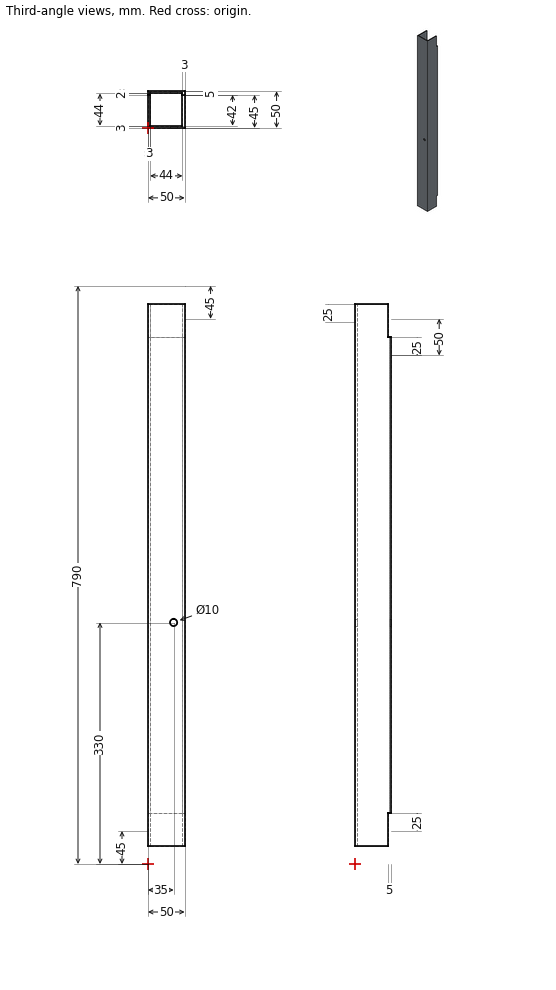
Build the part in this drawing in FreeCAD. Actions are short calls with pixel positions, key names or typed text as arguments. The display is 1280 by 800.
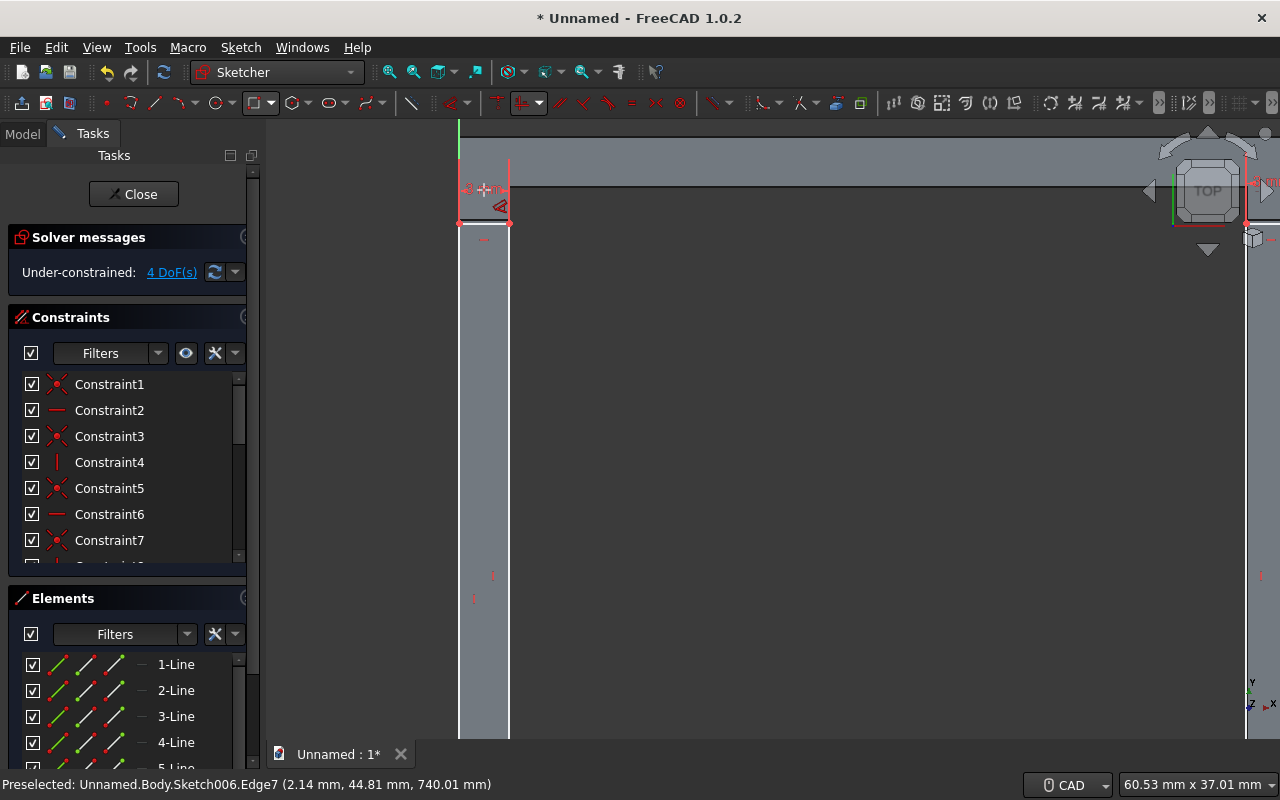
scroll(494, 224, down, 3)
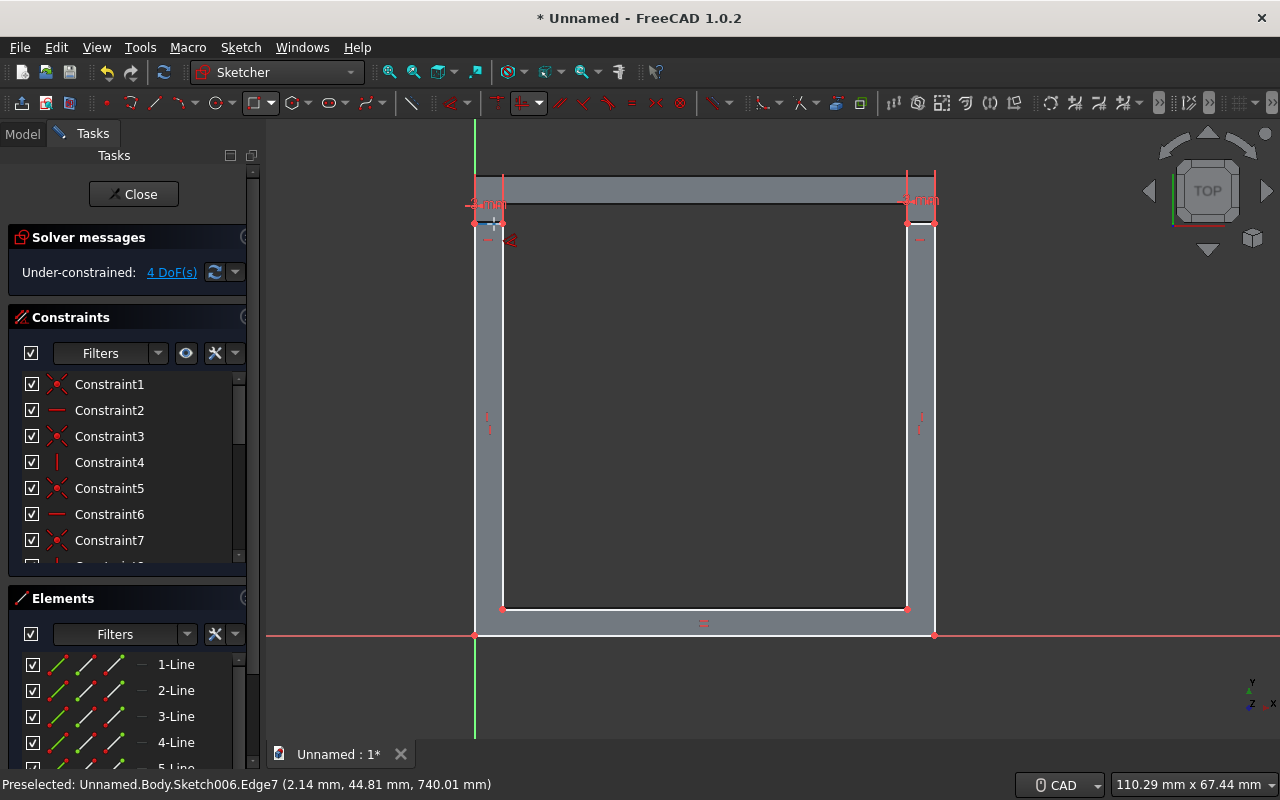
click(613, 636)
click(705, 670)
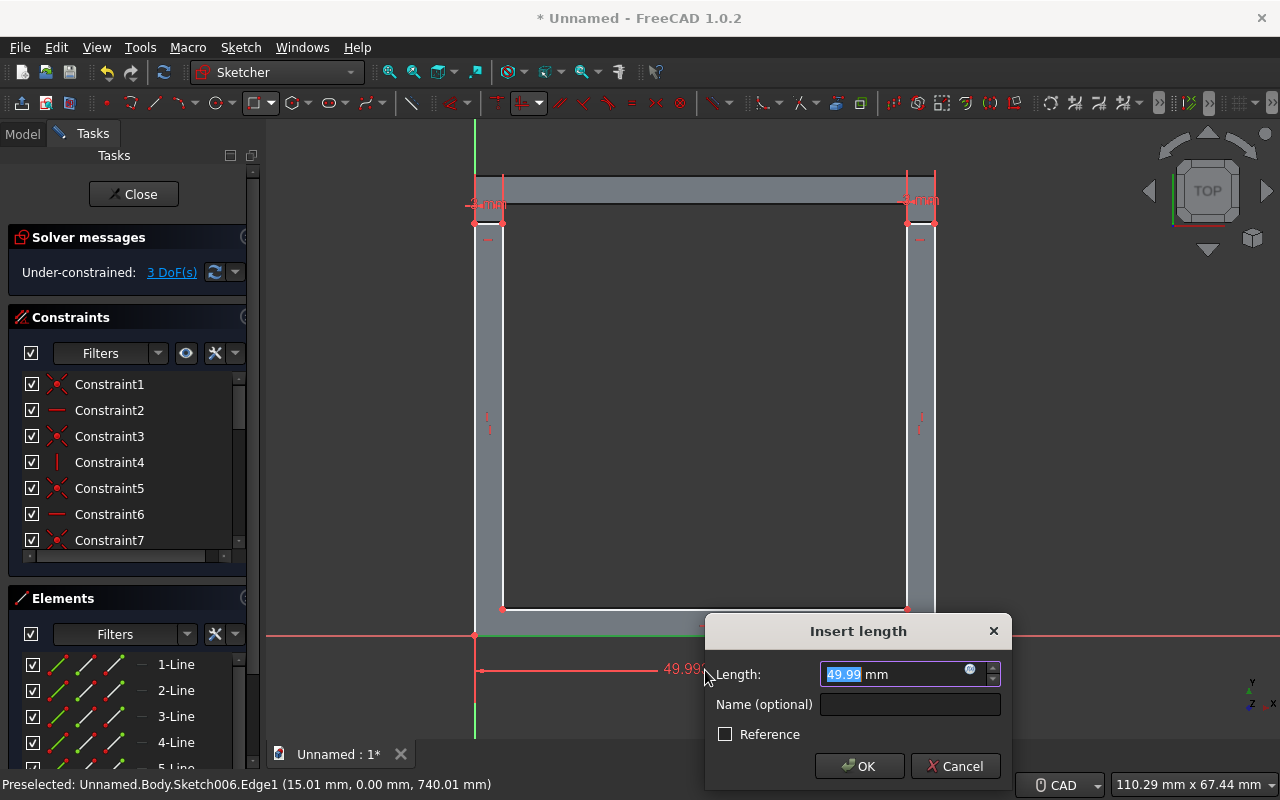
text(50)
key(Return)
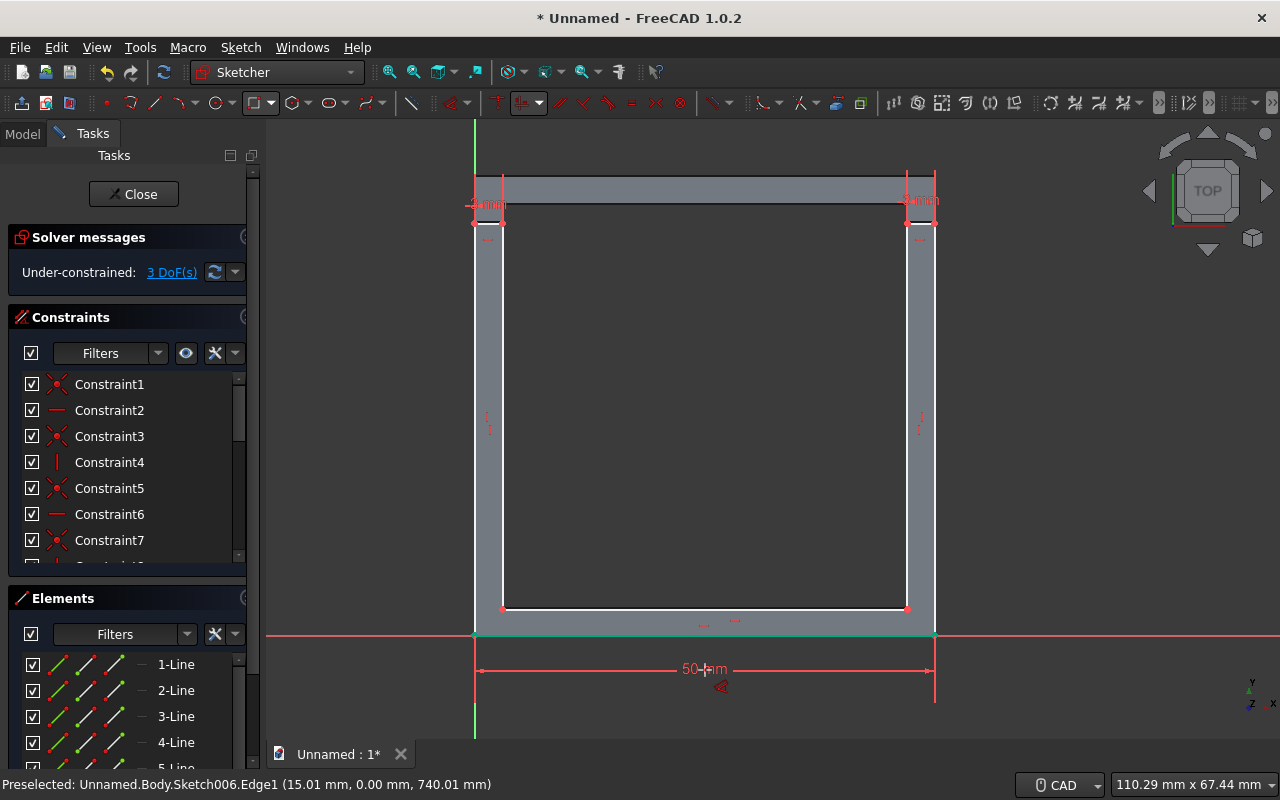
click(935, 512)
click(969, 430)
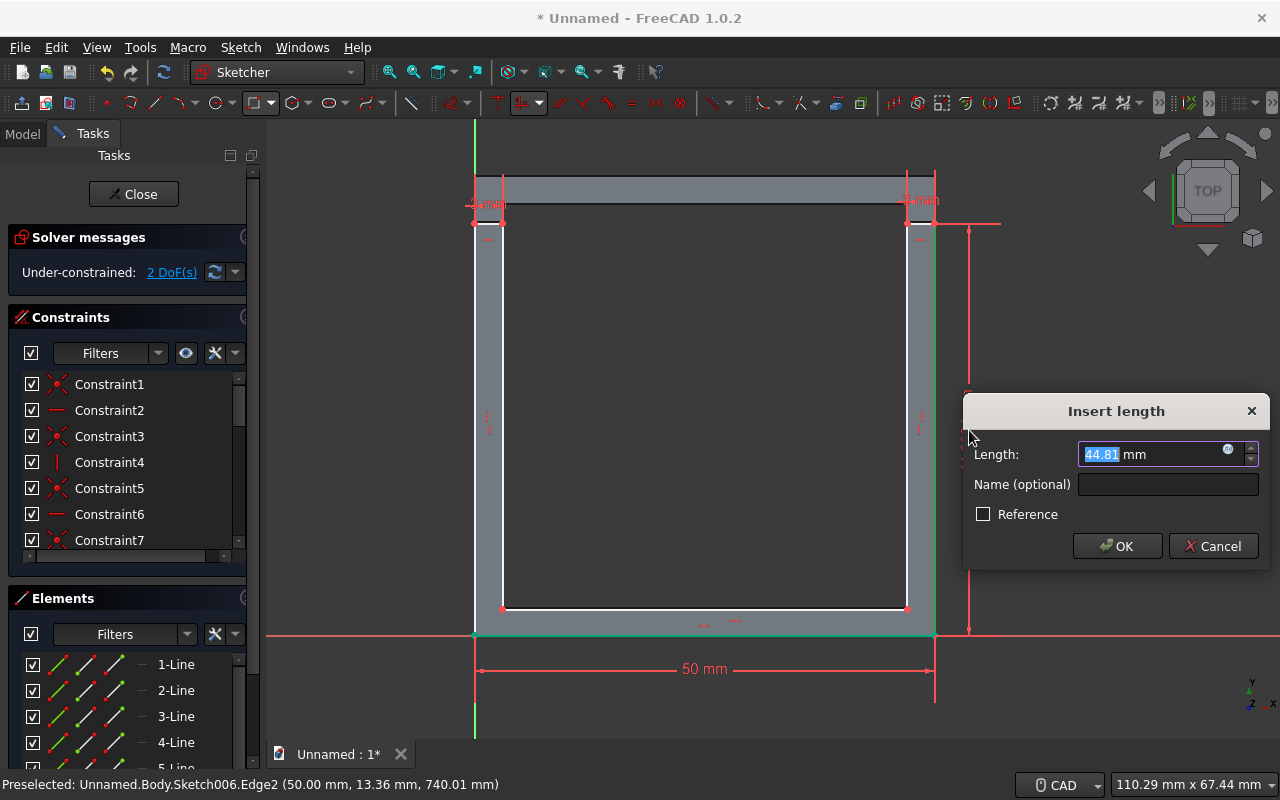
text(45)
key(Return)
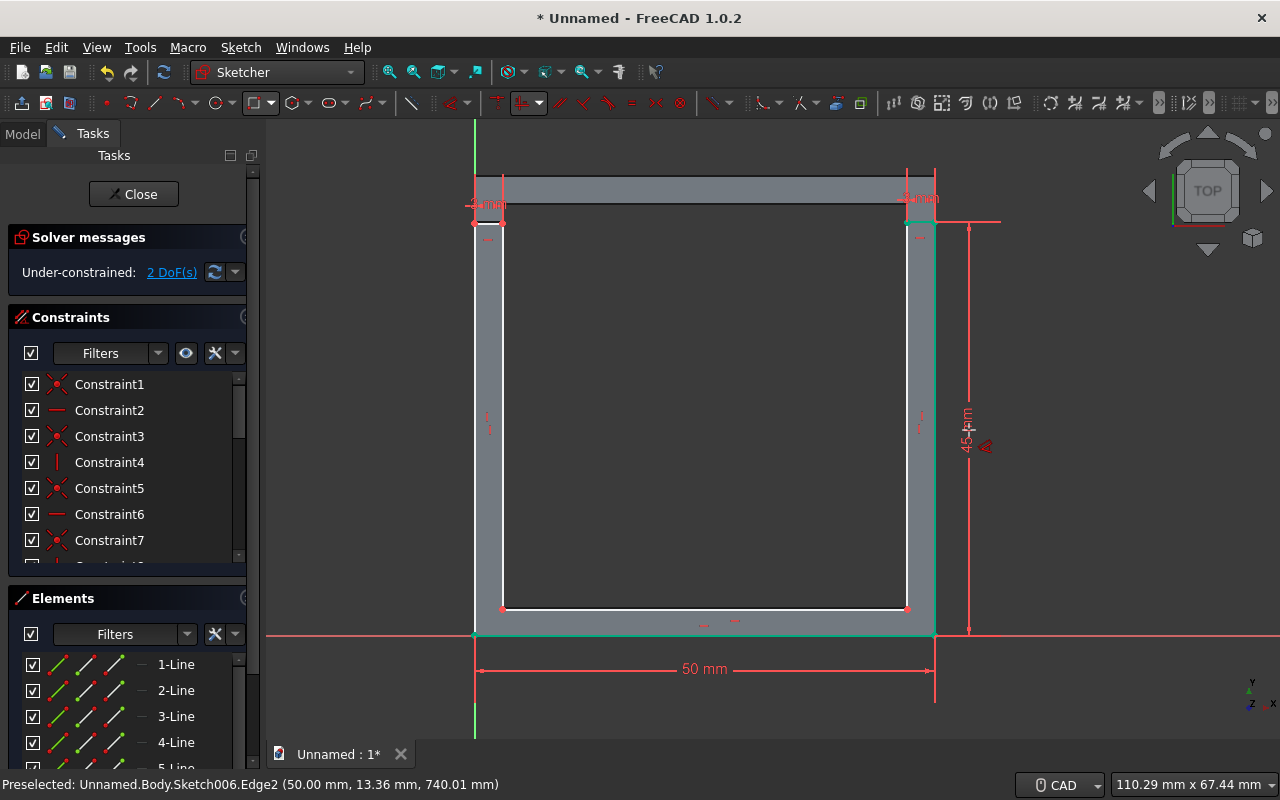
click(907, 338)
click(873, 416)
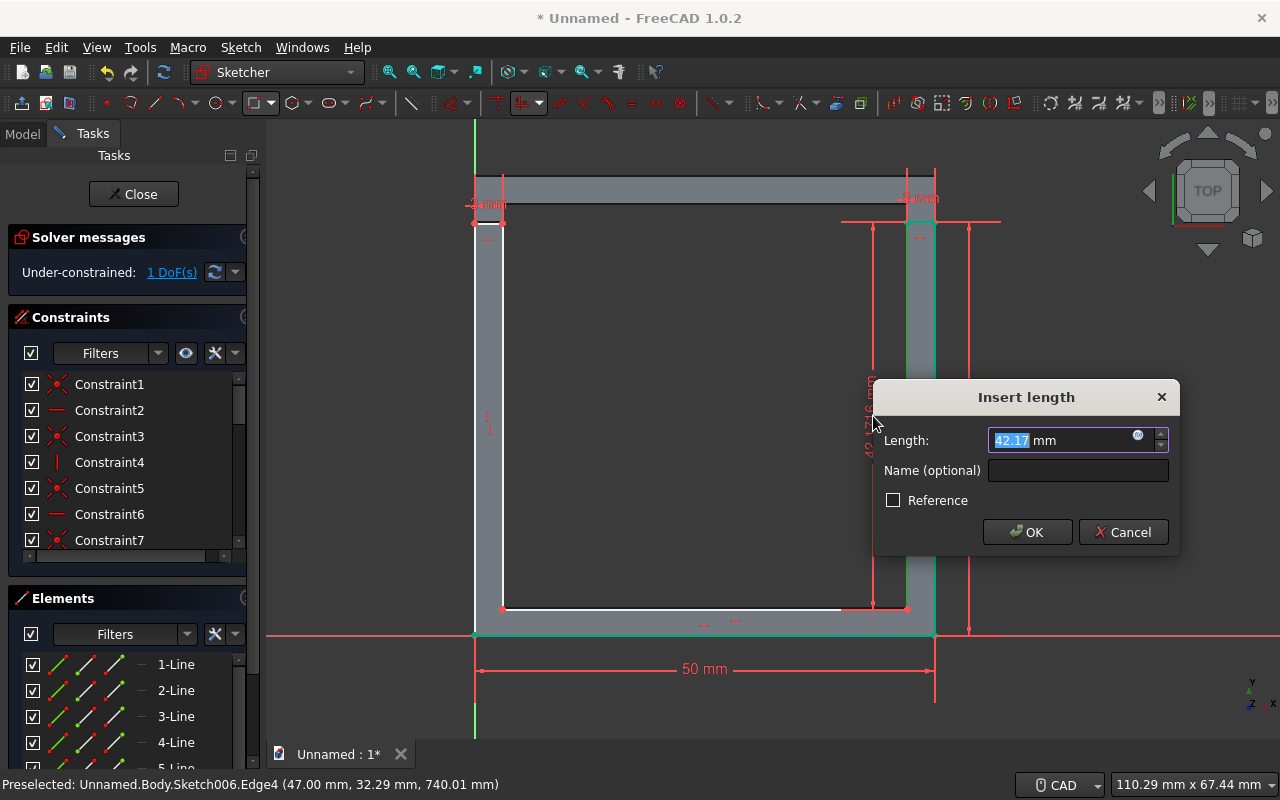
text(42)
key(Return)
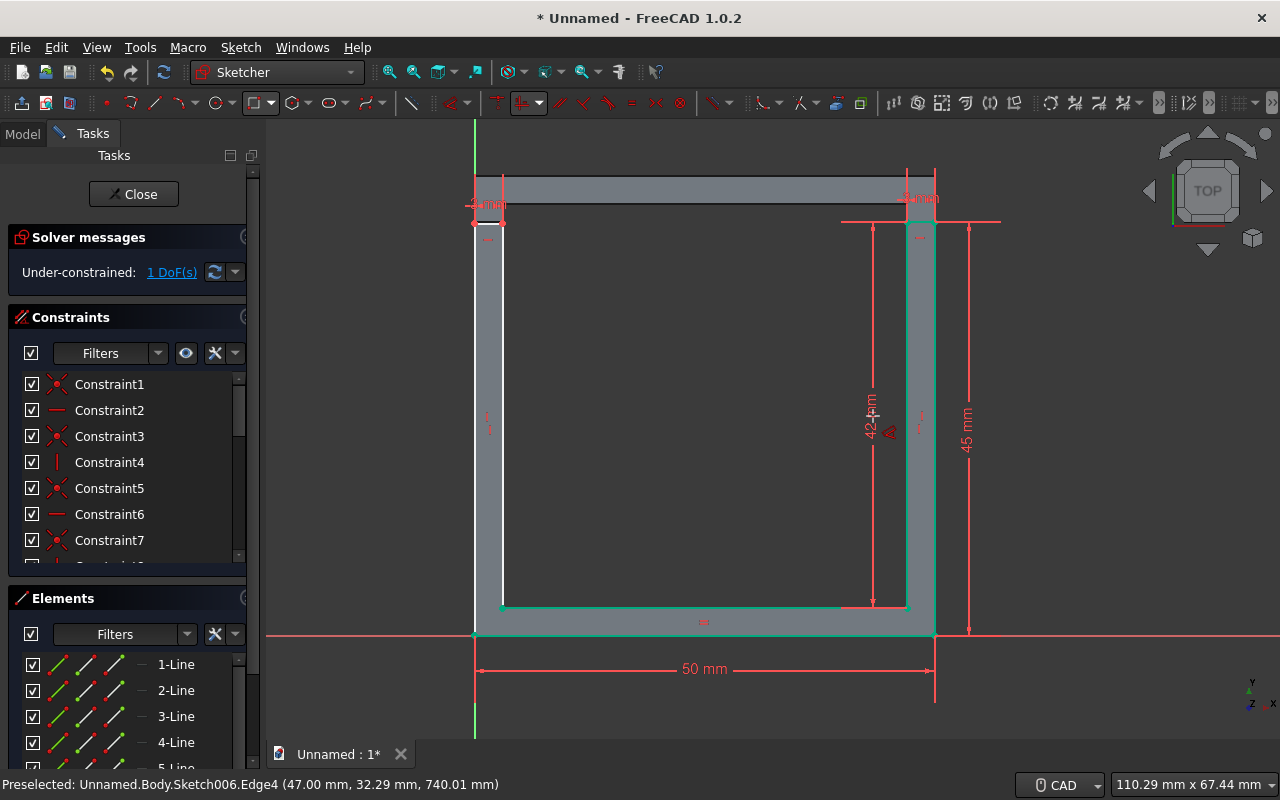
click(503, 493)
click(537, 416)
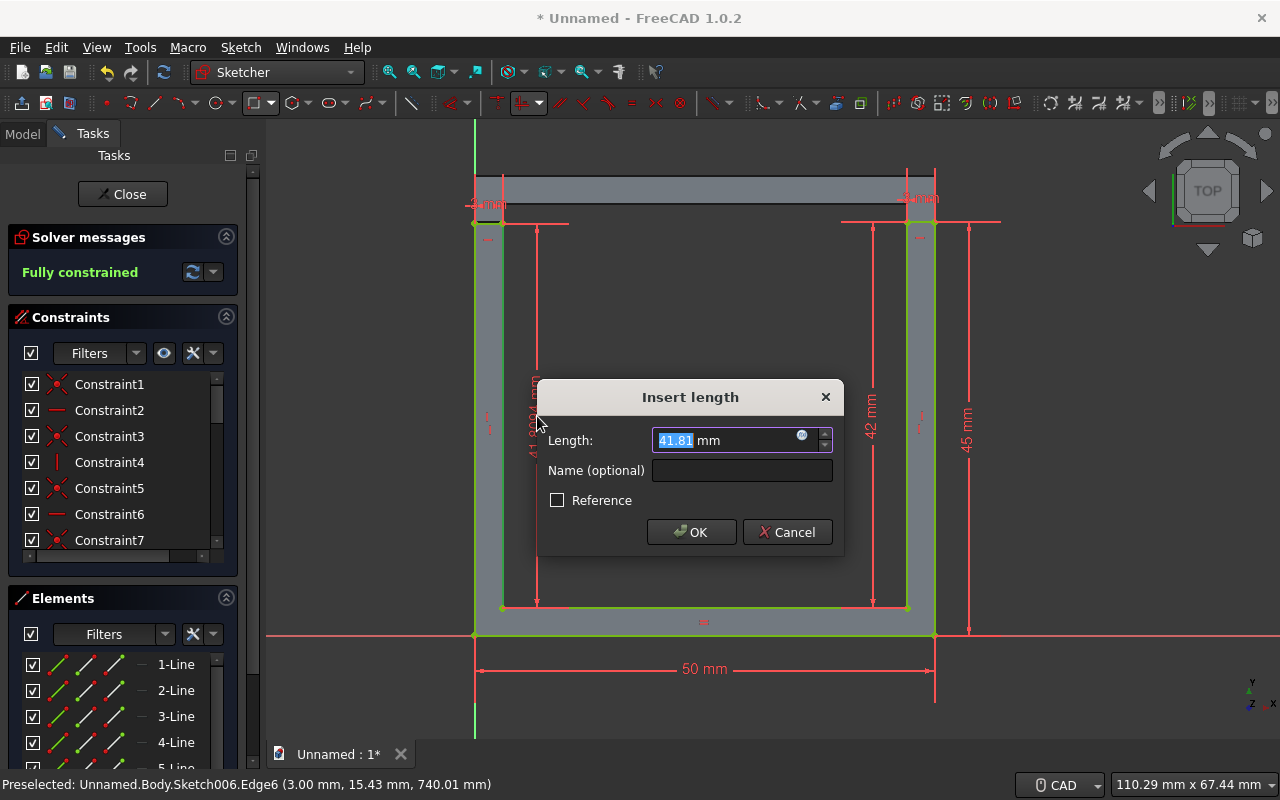
text(42)
key(Return)
key(Escape)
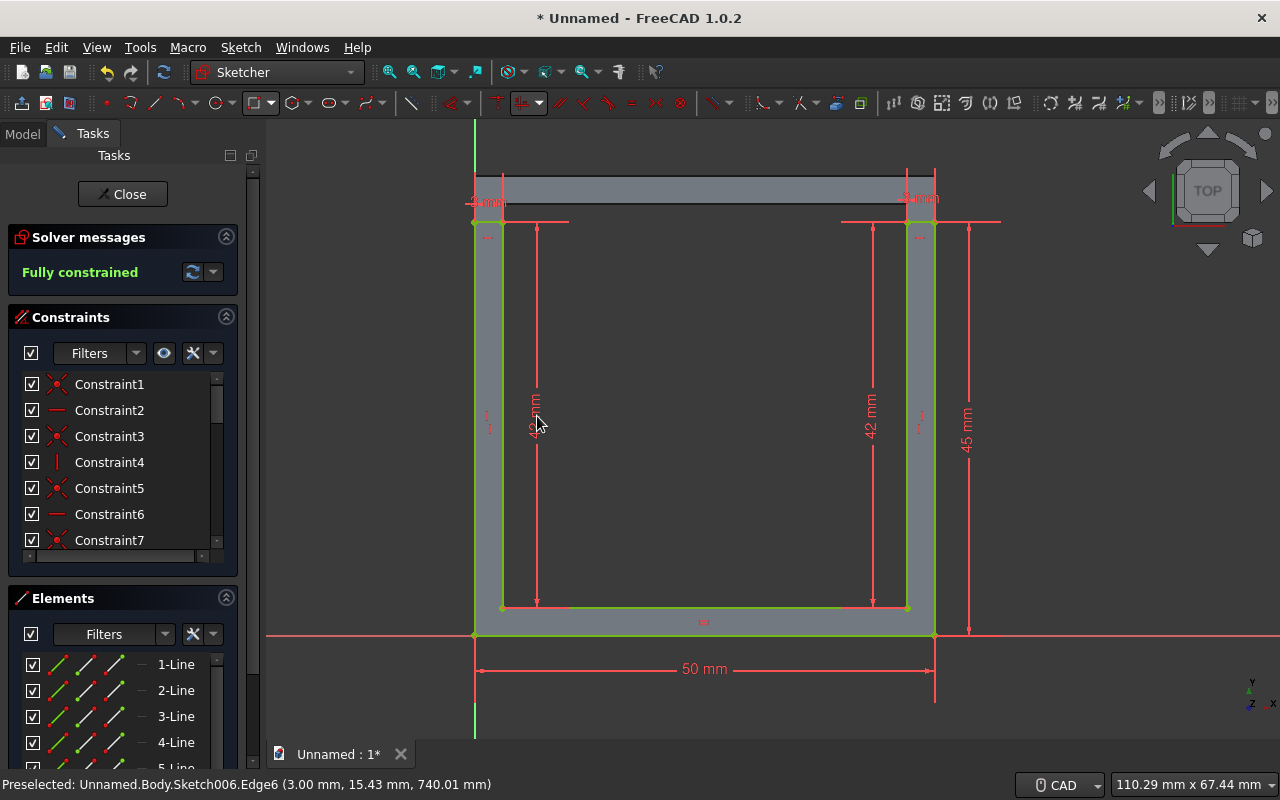
click(123, 194)